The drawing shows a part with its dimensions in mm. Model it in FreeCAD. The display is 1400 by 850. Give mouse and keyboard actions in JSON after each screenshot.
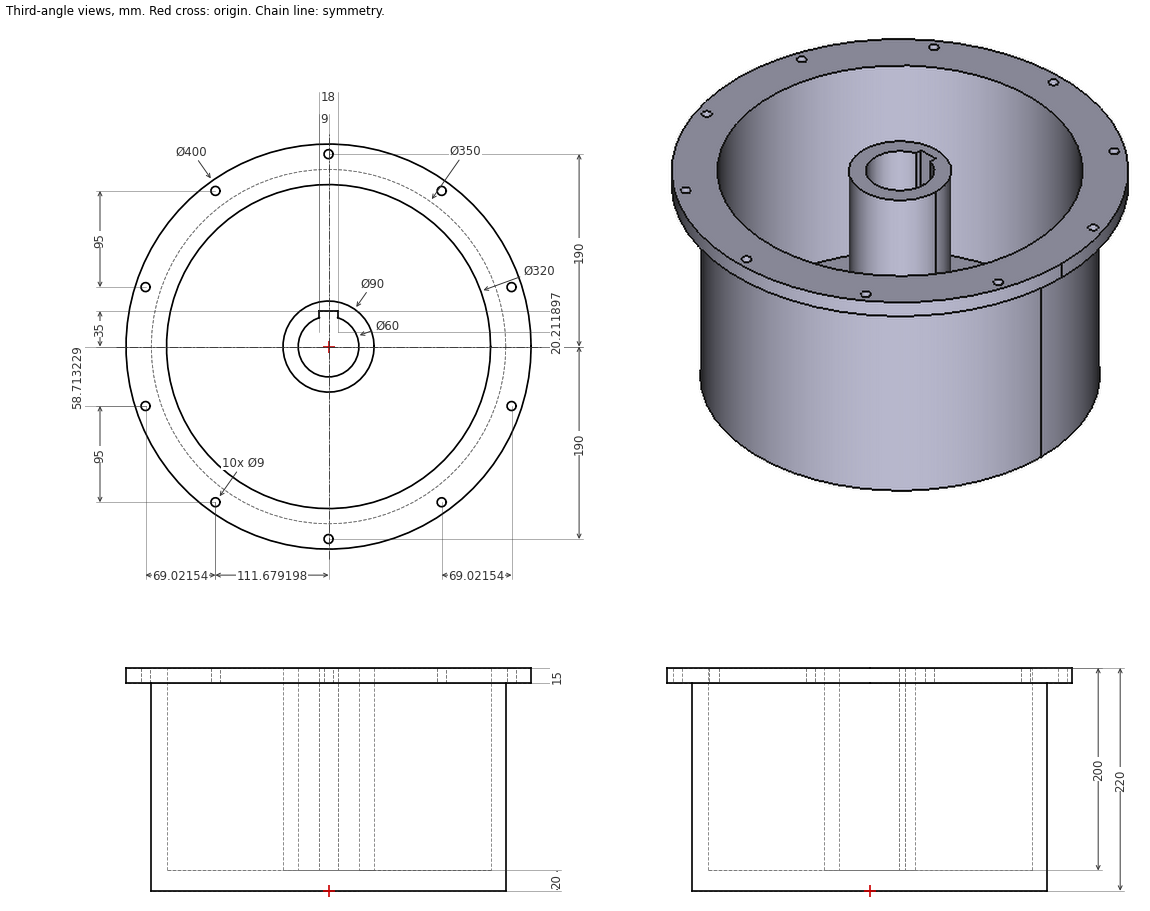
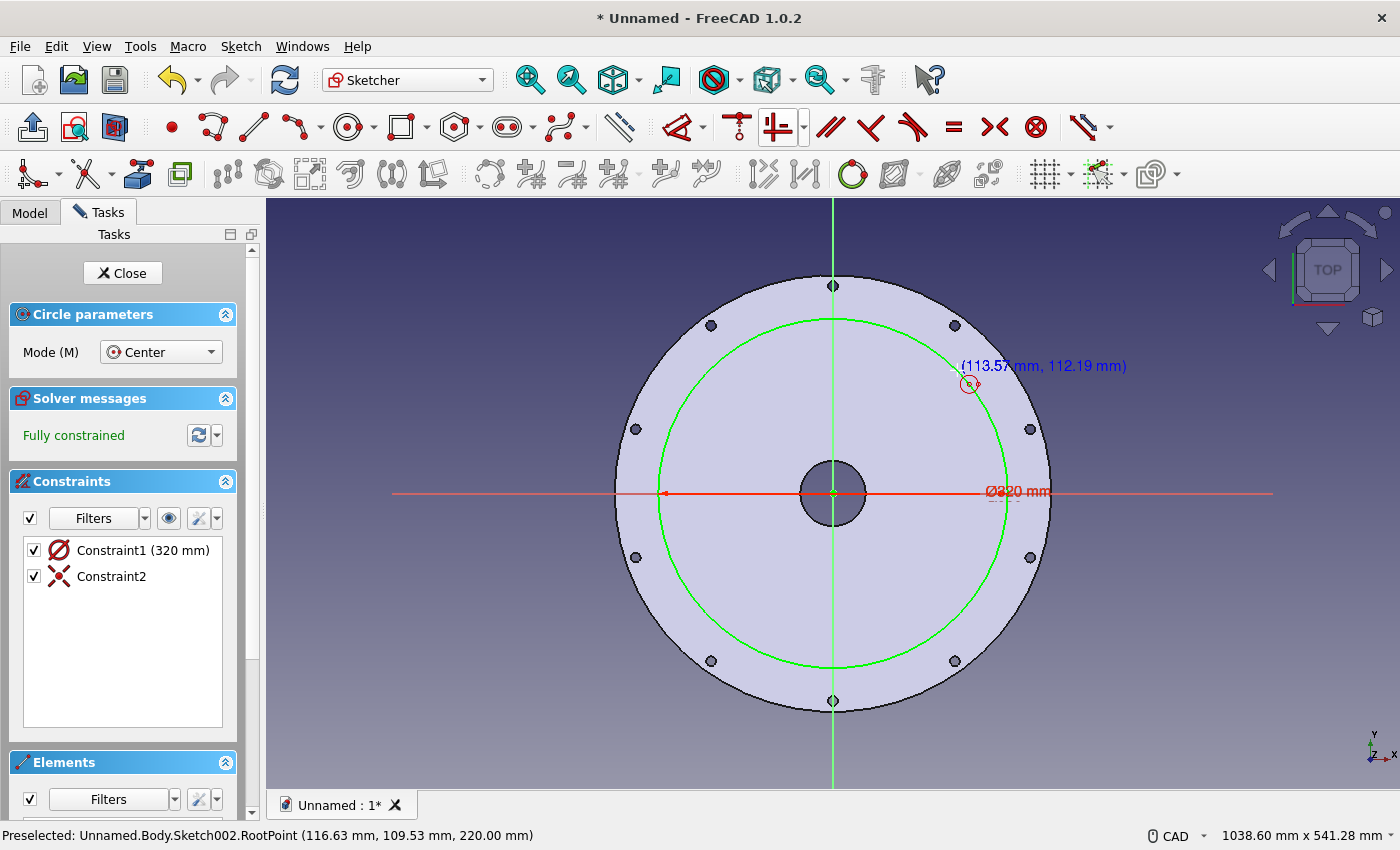
{"action": "left_click", "coordinate": [833, 494]}
{"action": "mouse_move", "coordinate": [868, 459]}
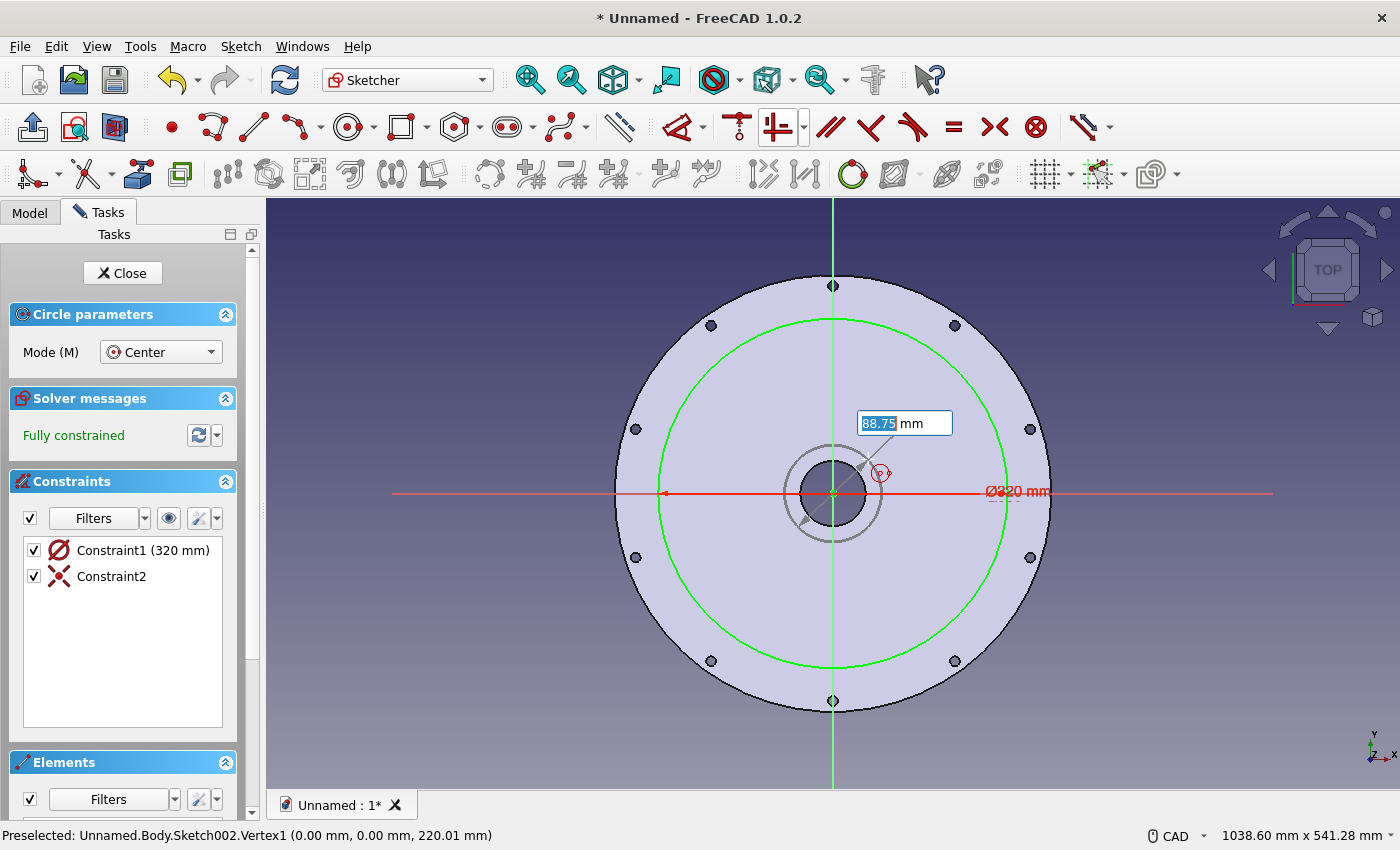
{"action": "type", "text": "90"}
{"action": "key", "text": "Return"}
{"action": "key", "text": "Escape"}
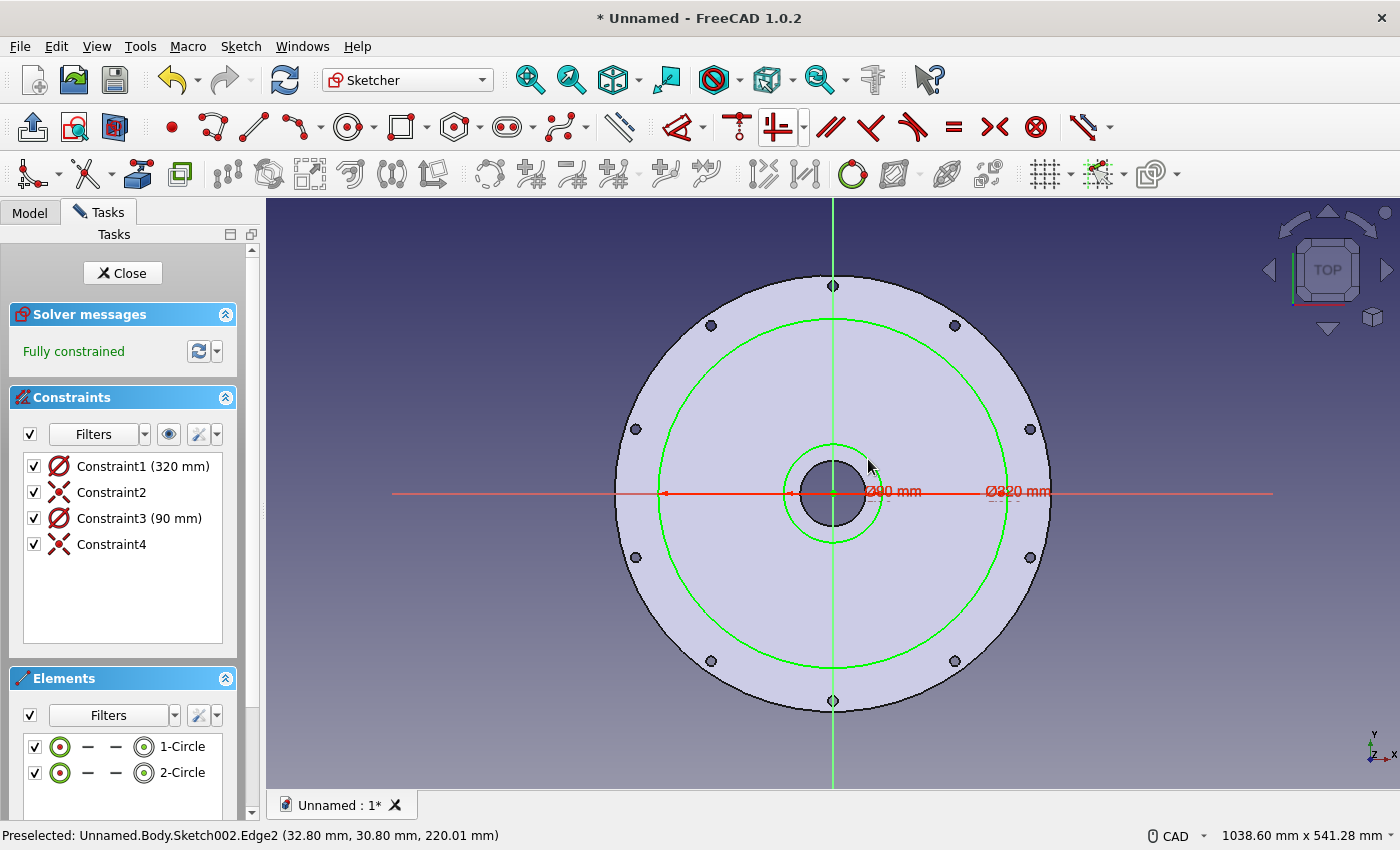
{"action": "left_click", "coordinate": [123, 273]}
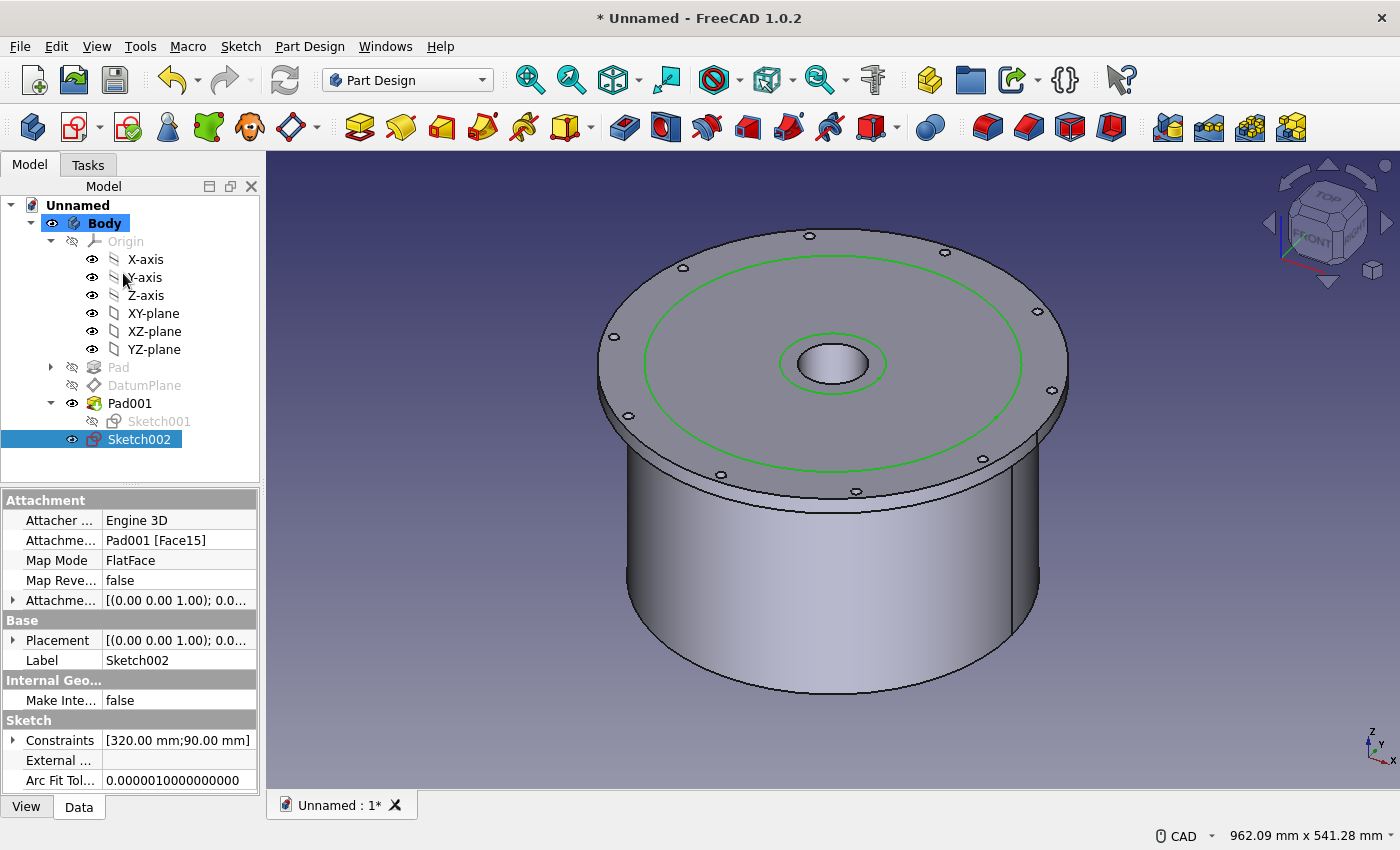
{"action": "left_click", "coordinate": [625, 128]}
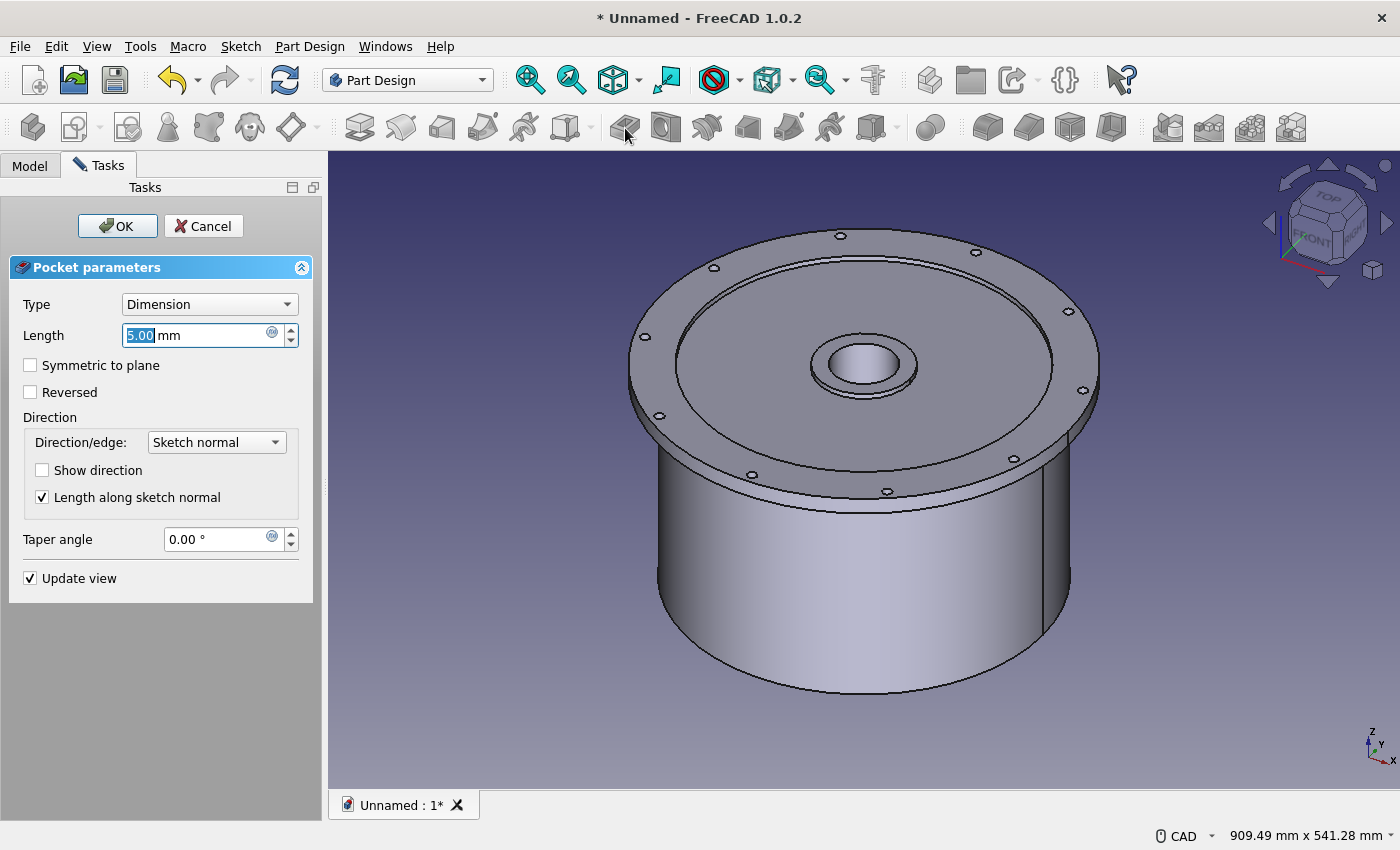
{"action": "type", "text": "200"}
{"action": "key", "text": "Tab"}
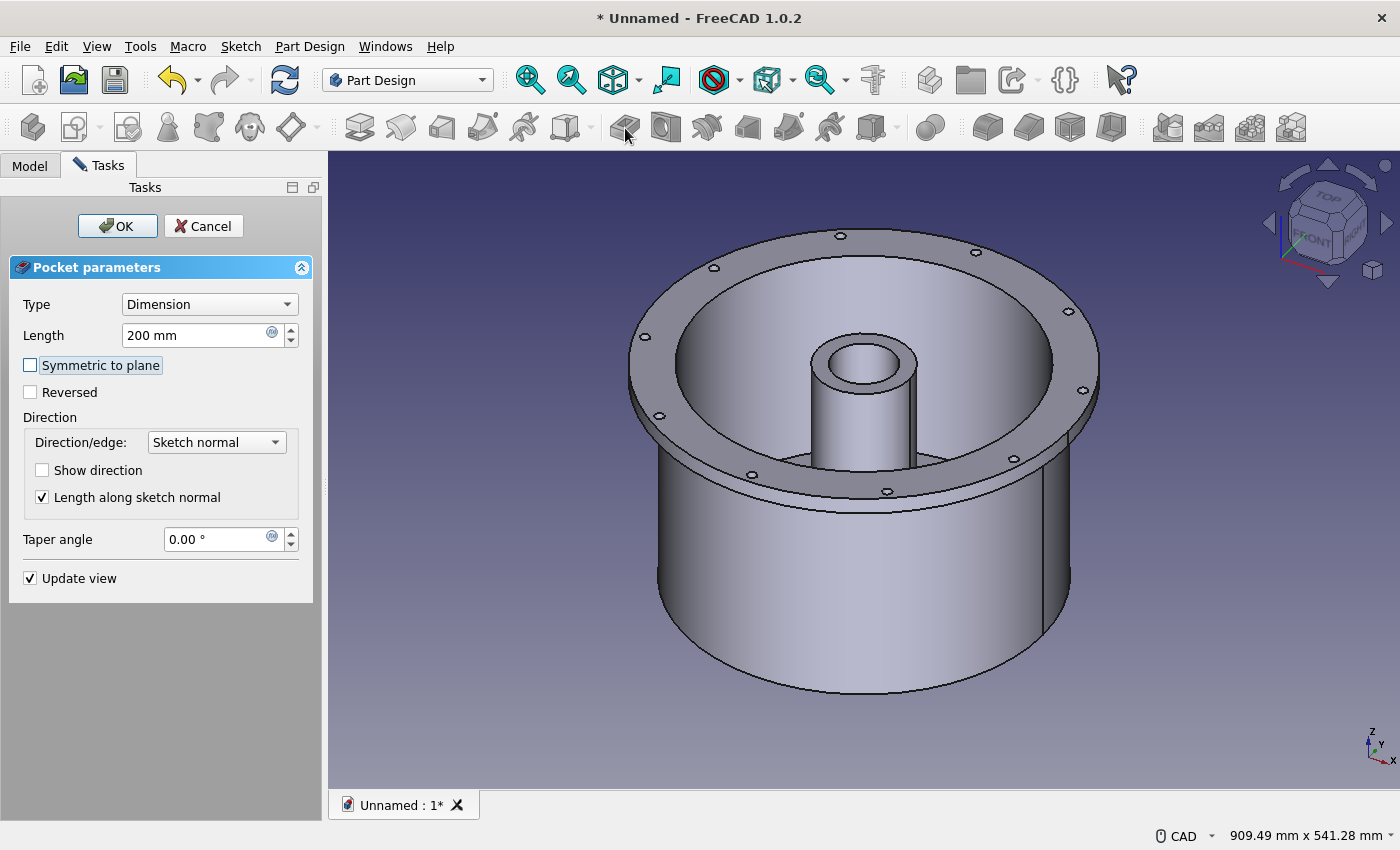
{"action": "left_click", "coordinate": [118, 226]}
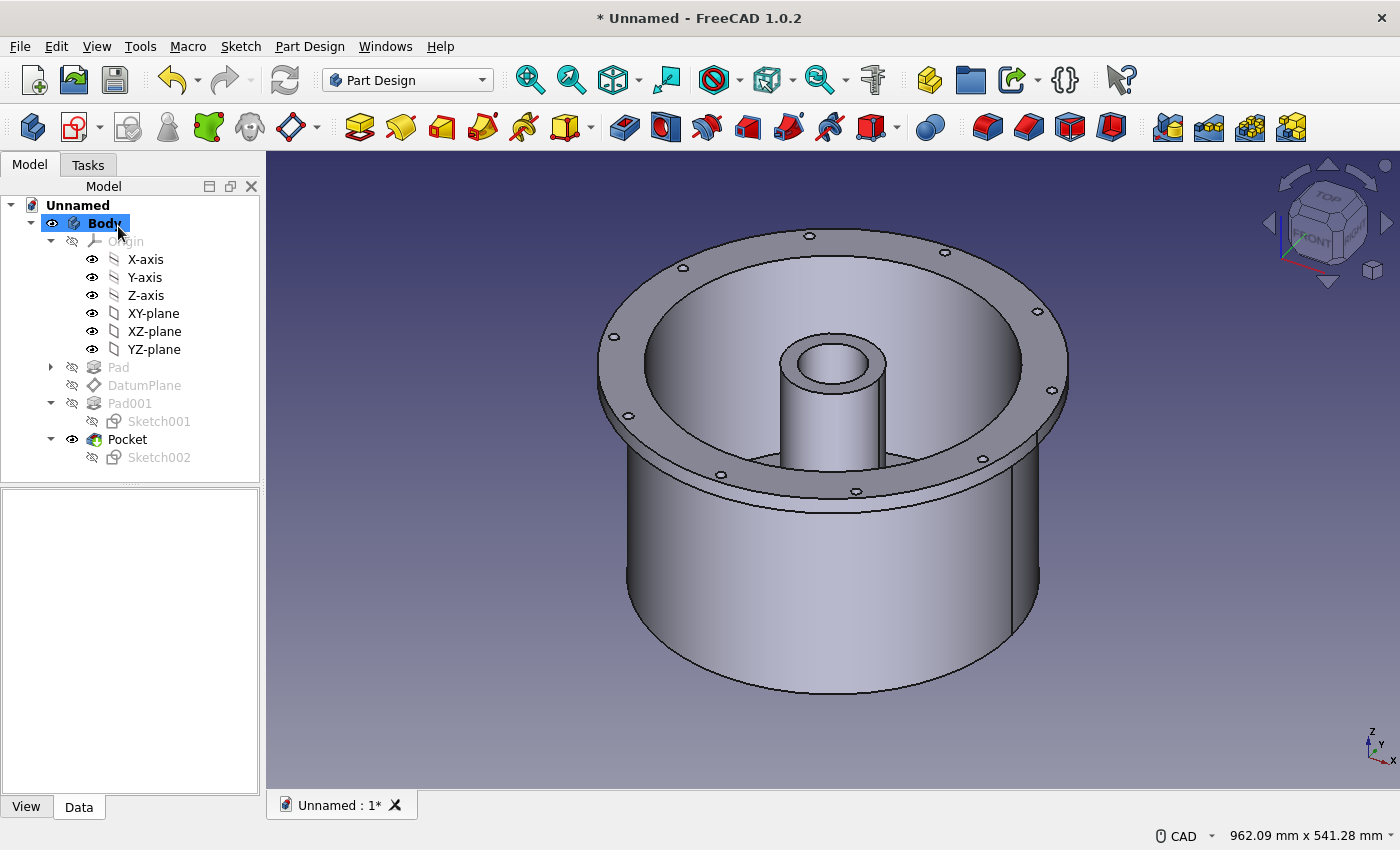
{"action": "left_click", "coordinate": [74, 128]}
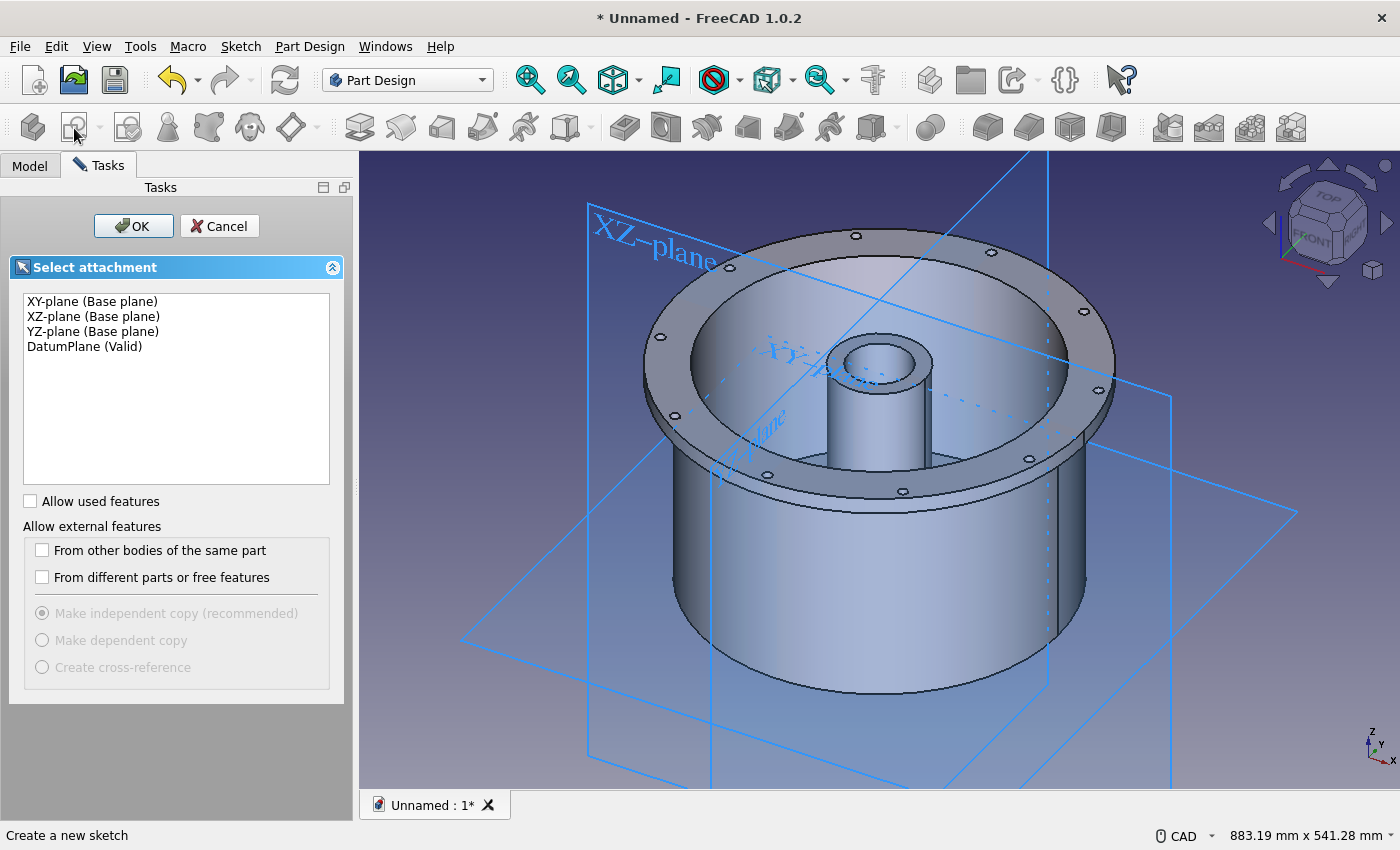
{"action": "left_click", "coordinate": [84, 302]}